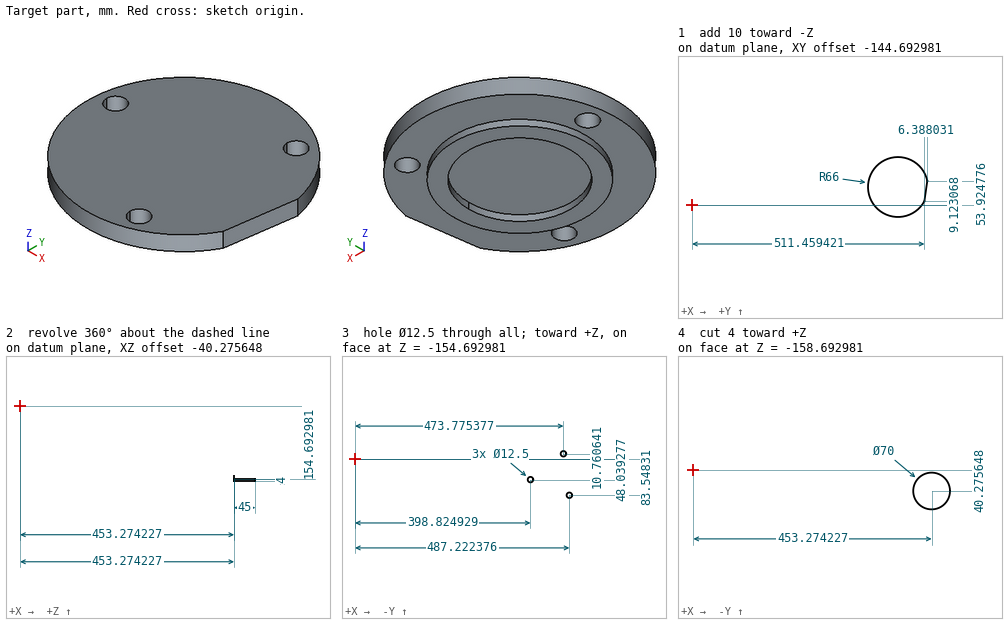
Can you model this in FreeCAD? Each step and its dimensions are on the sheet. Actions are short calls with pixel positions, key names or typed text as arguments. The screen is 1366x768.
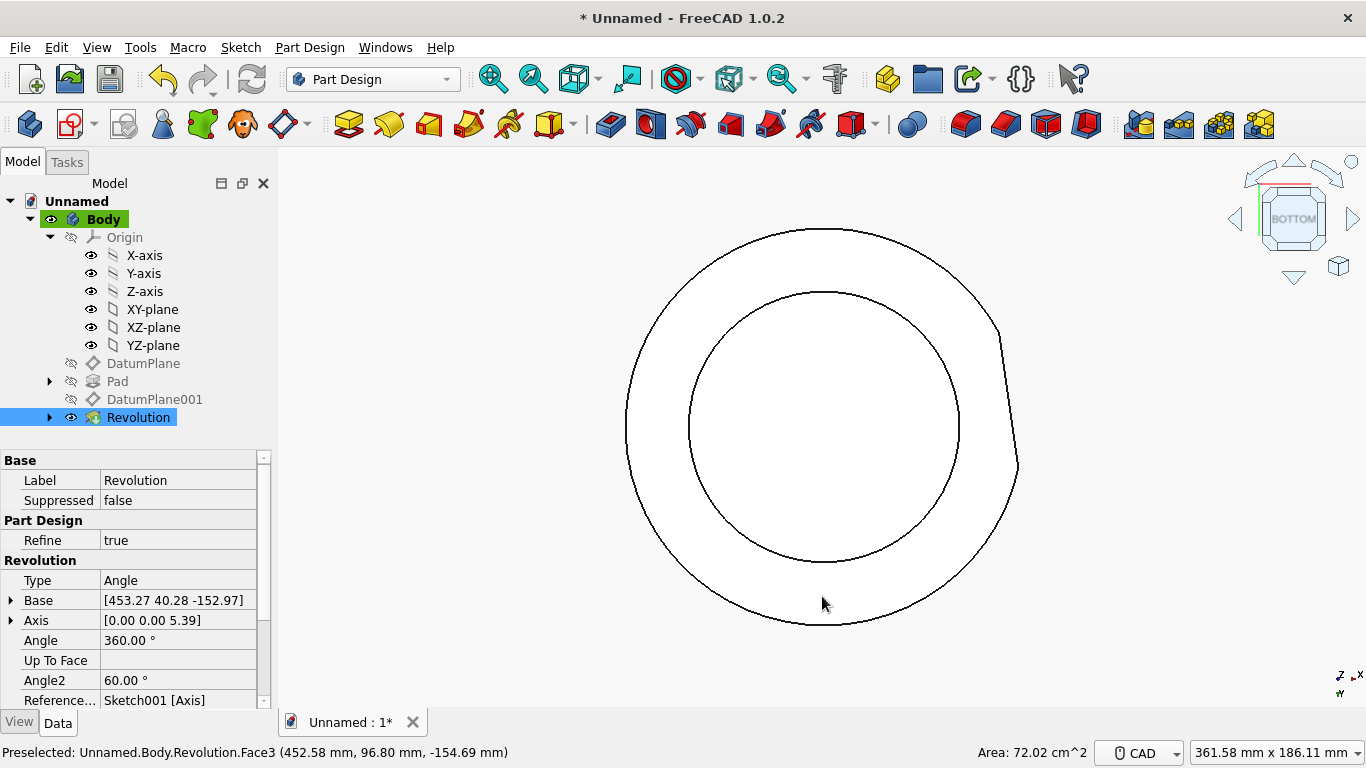
click(70, 124)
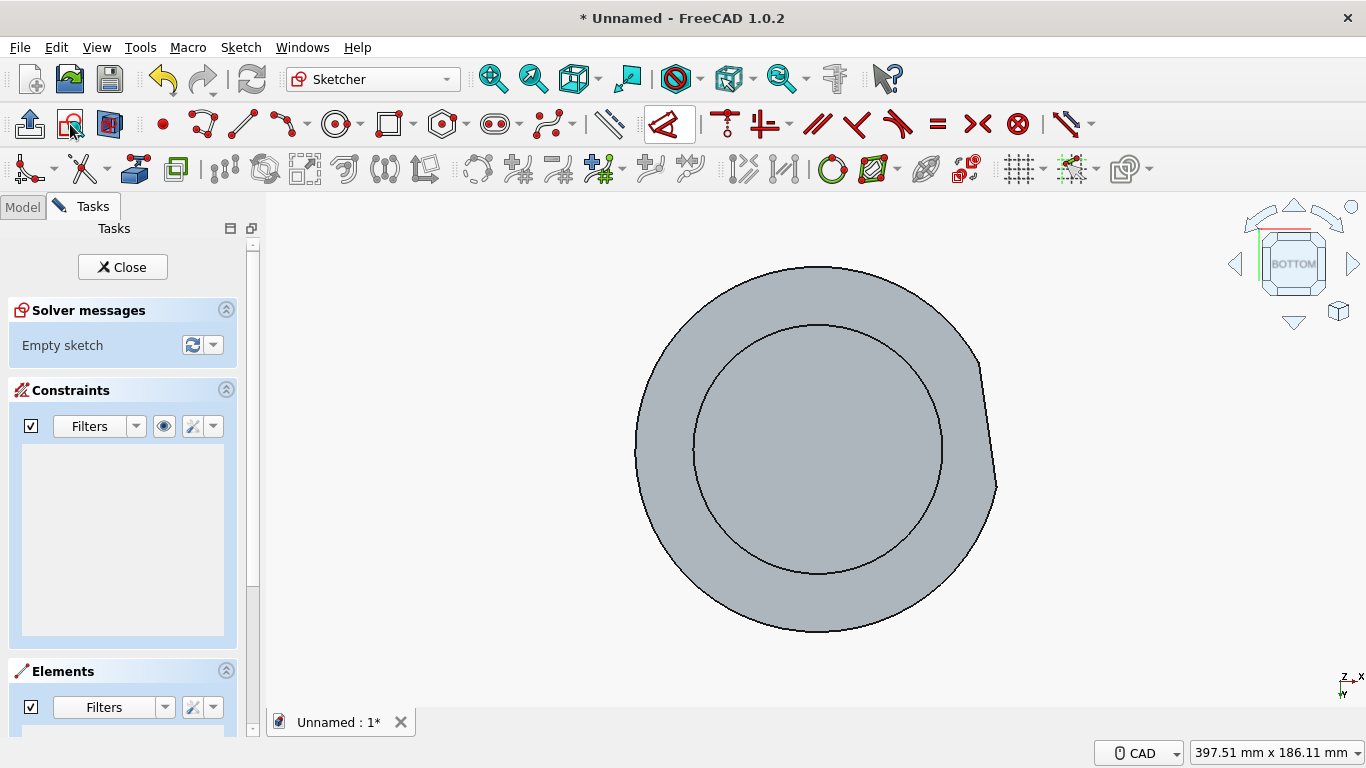
key(g)
key(c)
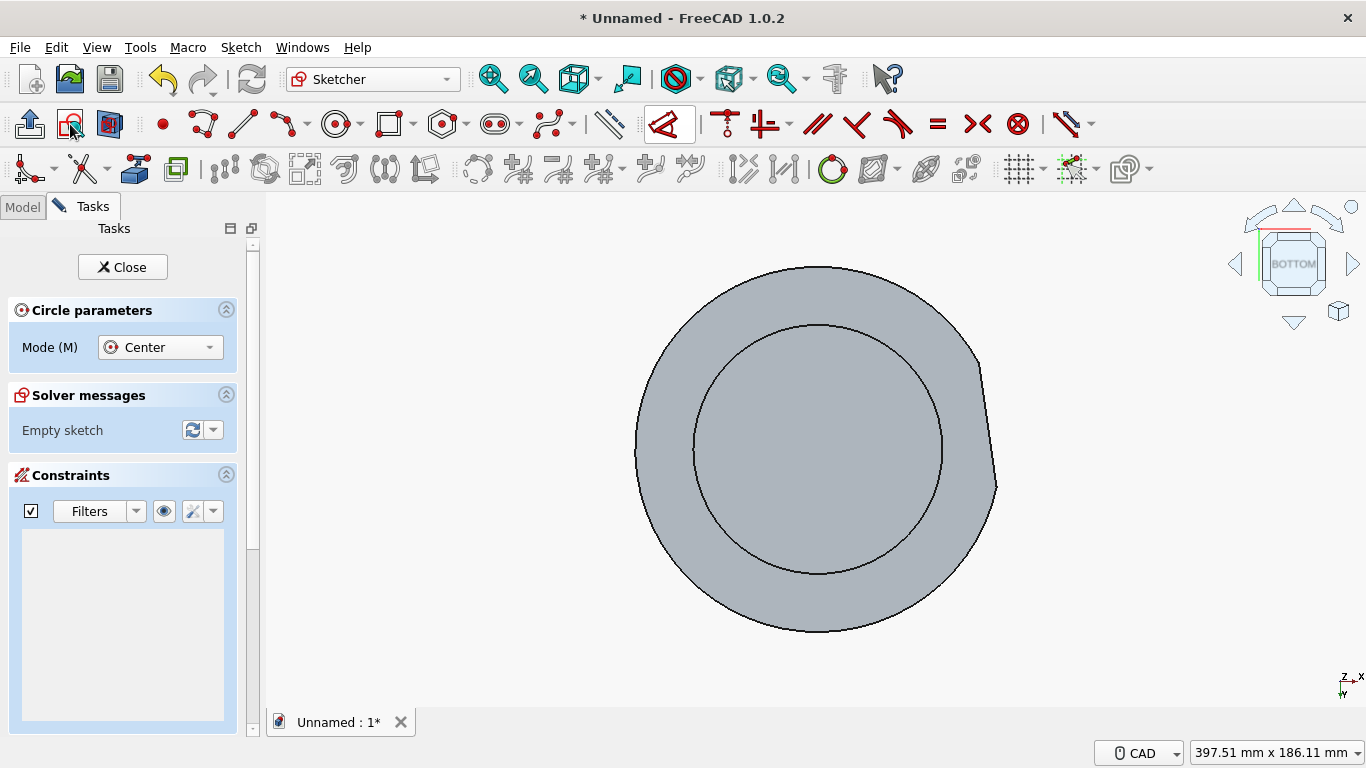
scroll(667, 471, up, 2)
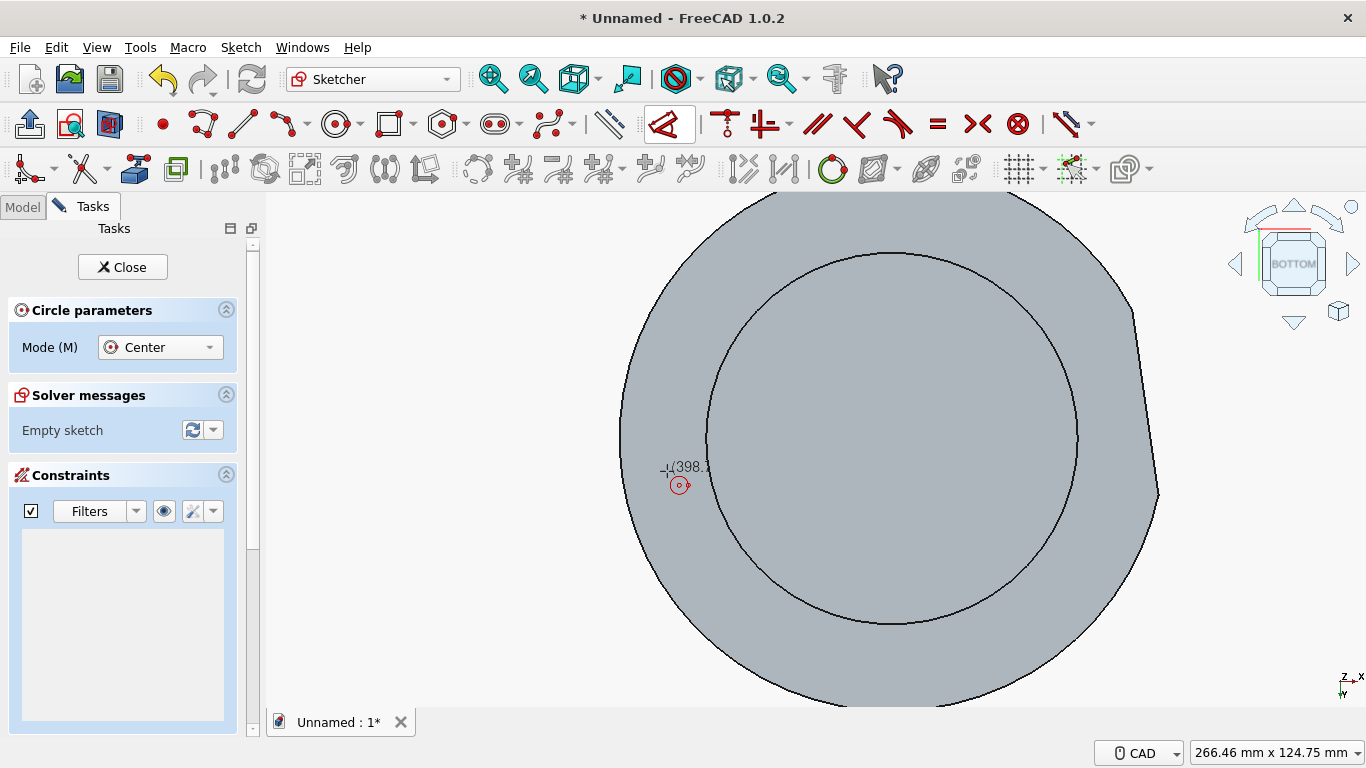
click(667, 471)
move(685, 452)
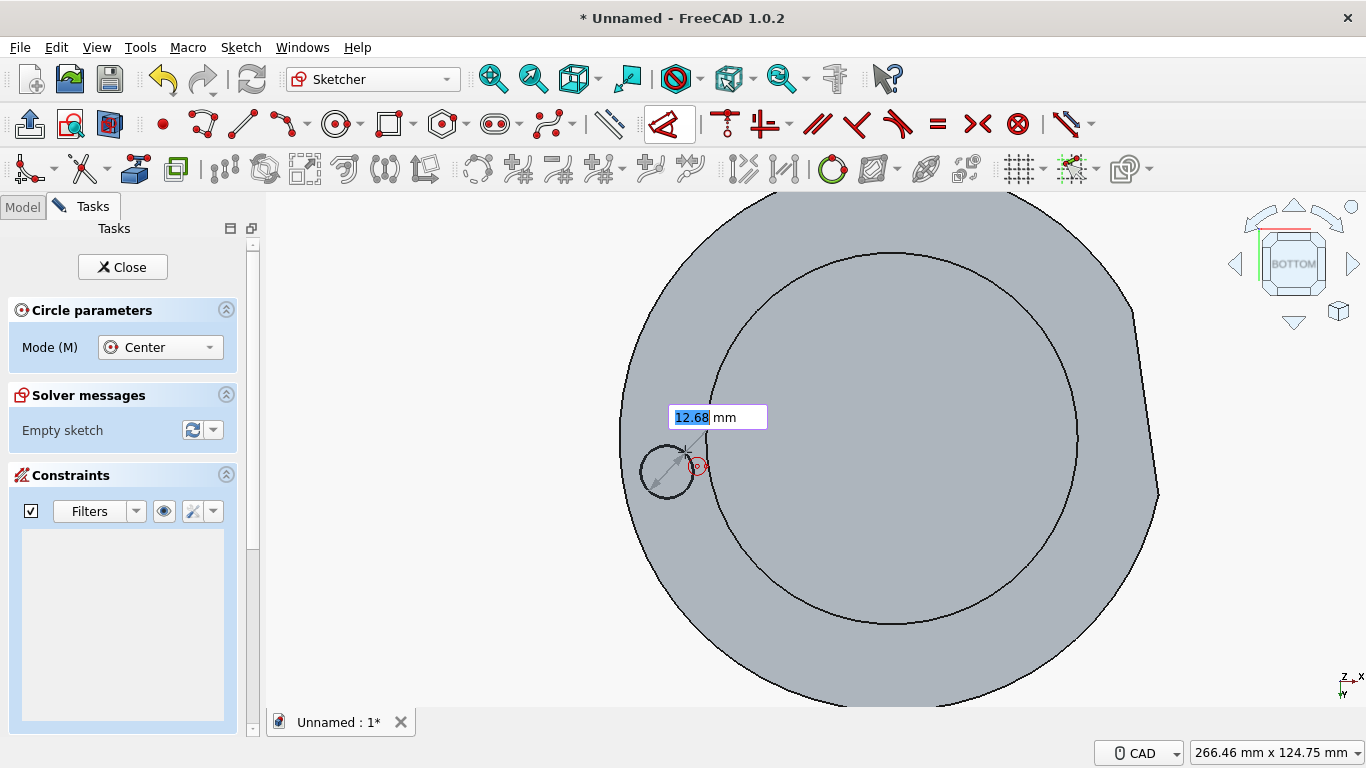
text(12.5)
key(Return)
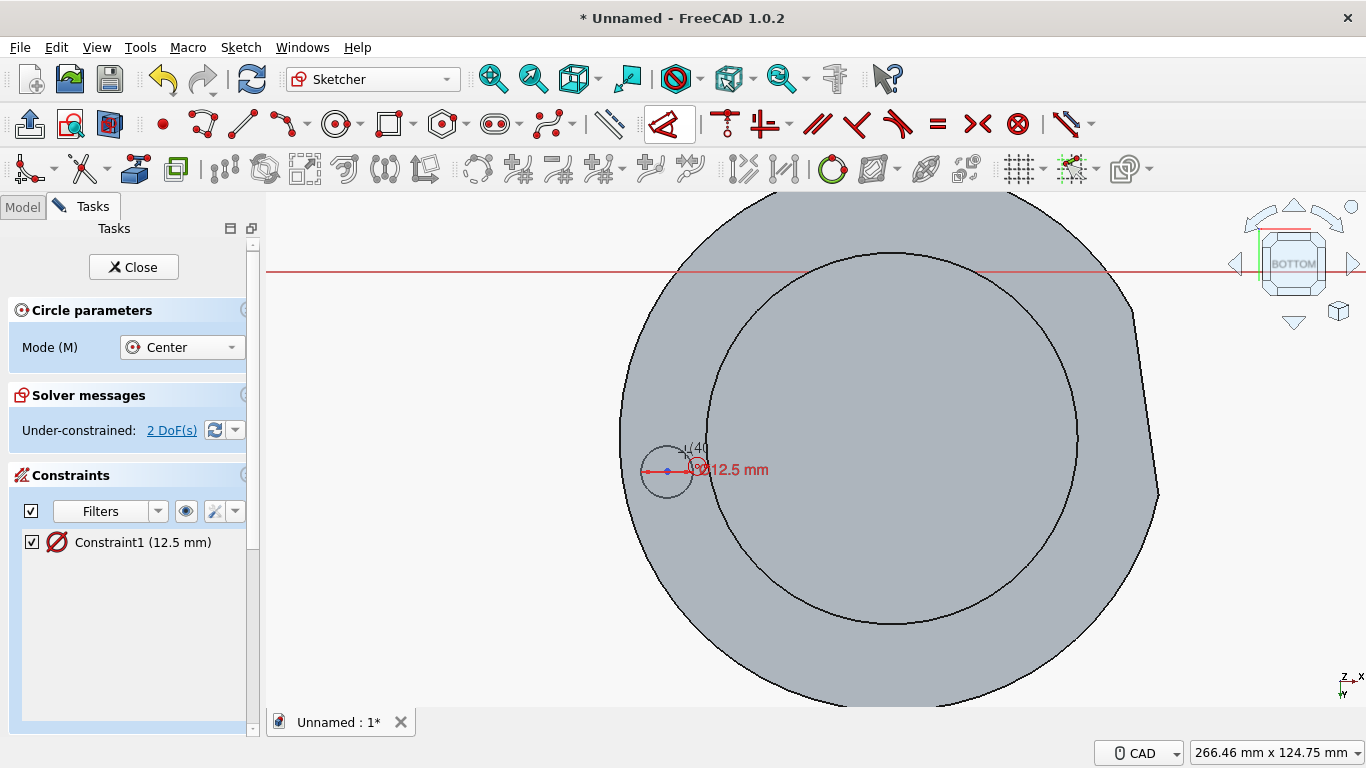
click(1032, 617)
move(1050, 599)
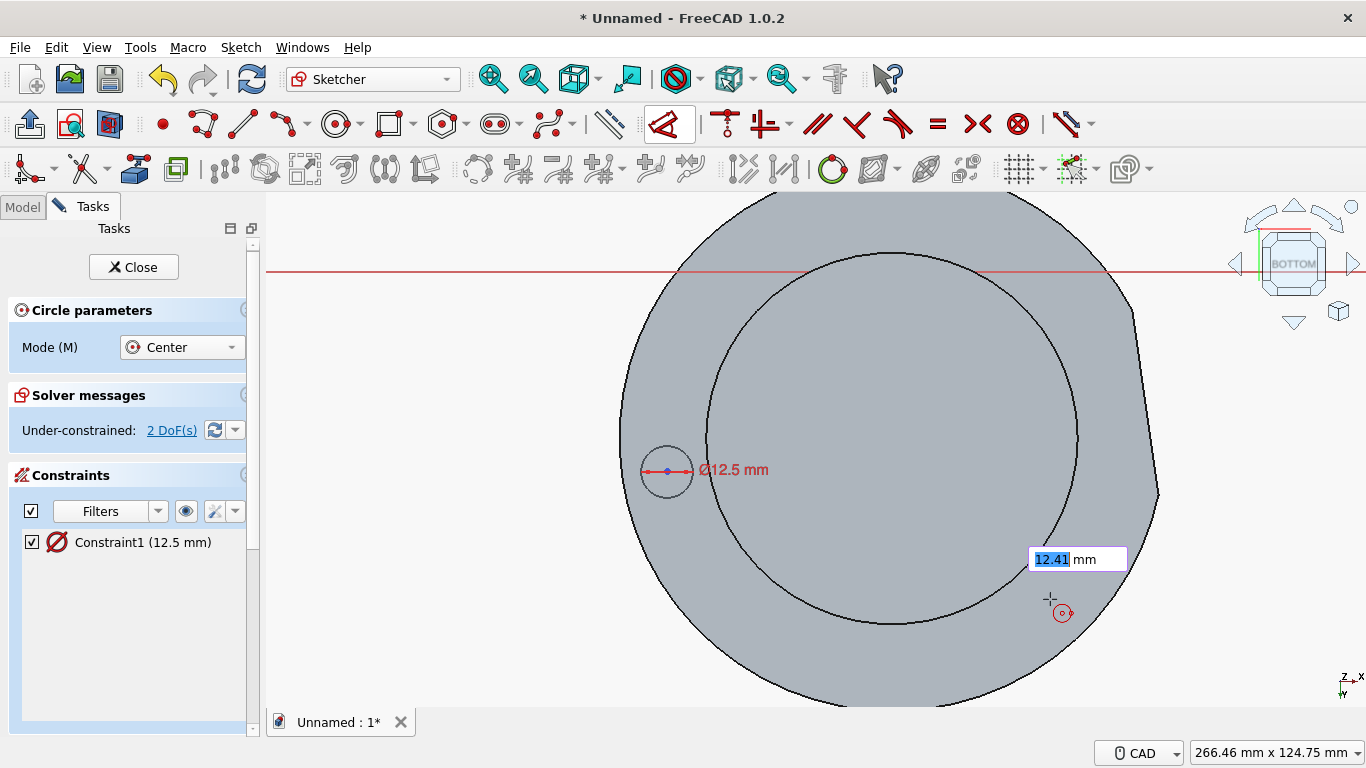
text(12.5)
key(Return)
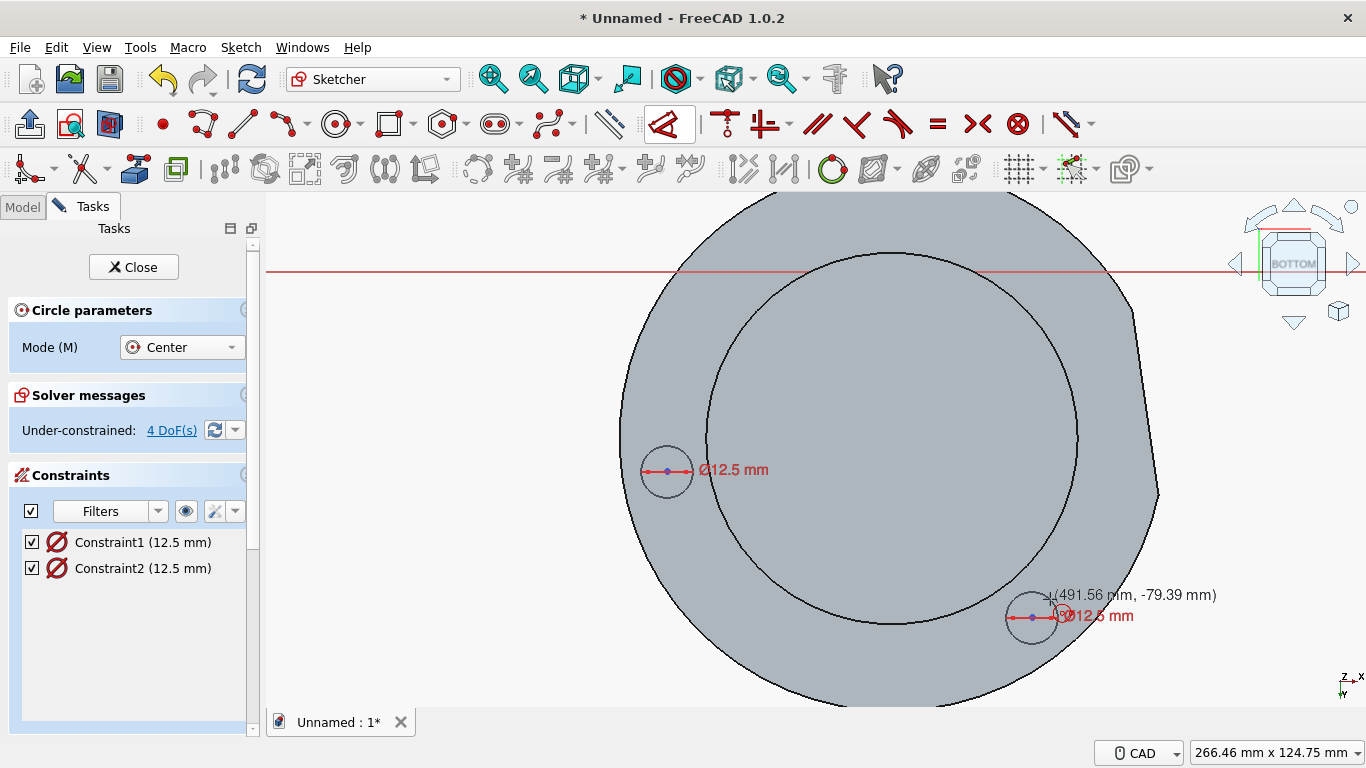
click(977, 228)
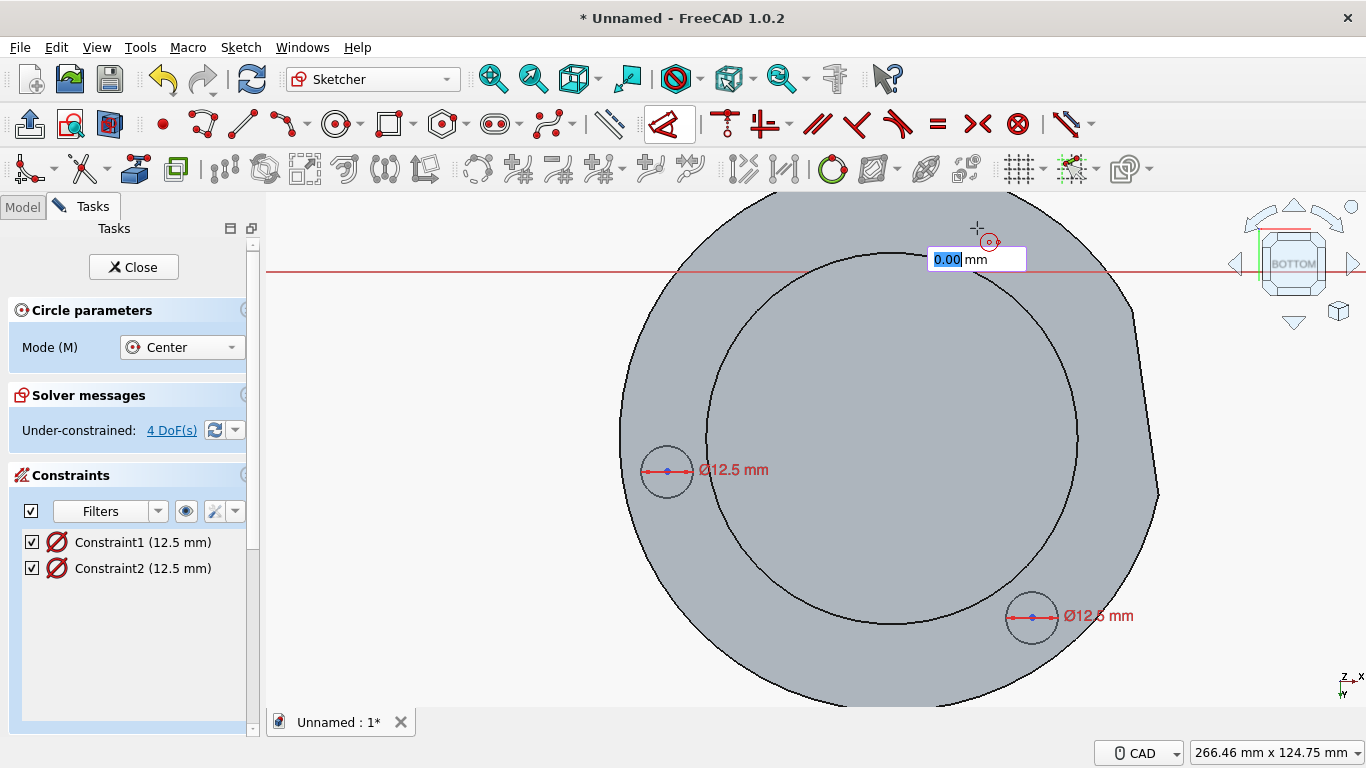
scroll(540, 504, down, 2)
move(845, 307)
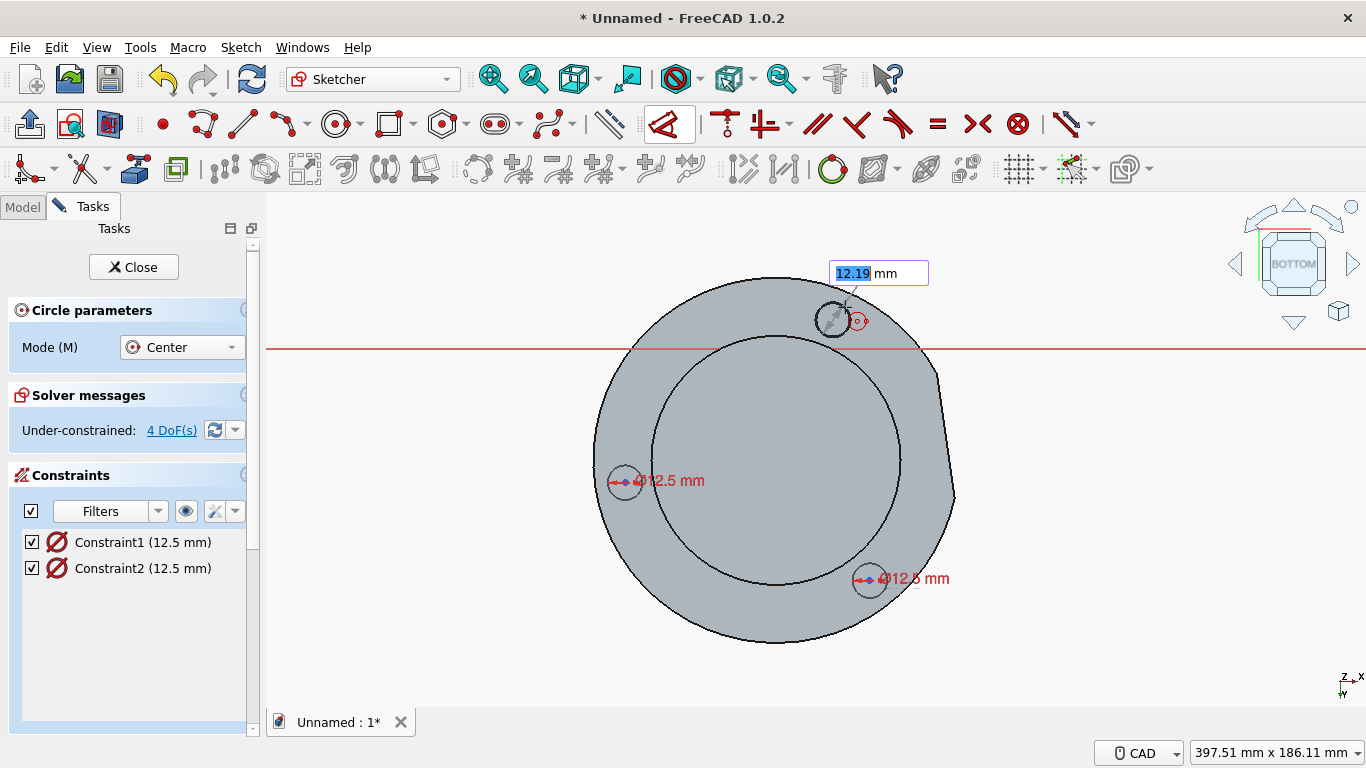
text(12.5)
key(Return)
key(Escape)